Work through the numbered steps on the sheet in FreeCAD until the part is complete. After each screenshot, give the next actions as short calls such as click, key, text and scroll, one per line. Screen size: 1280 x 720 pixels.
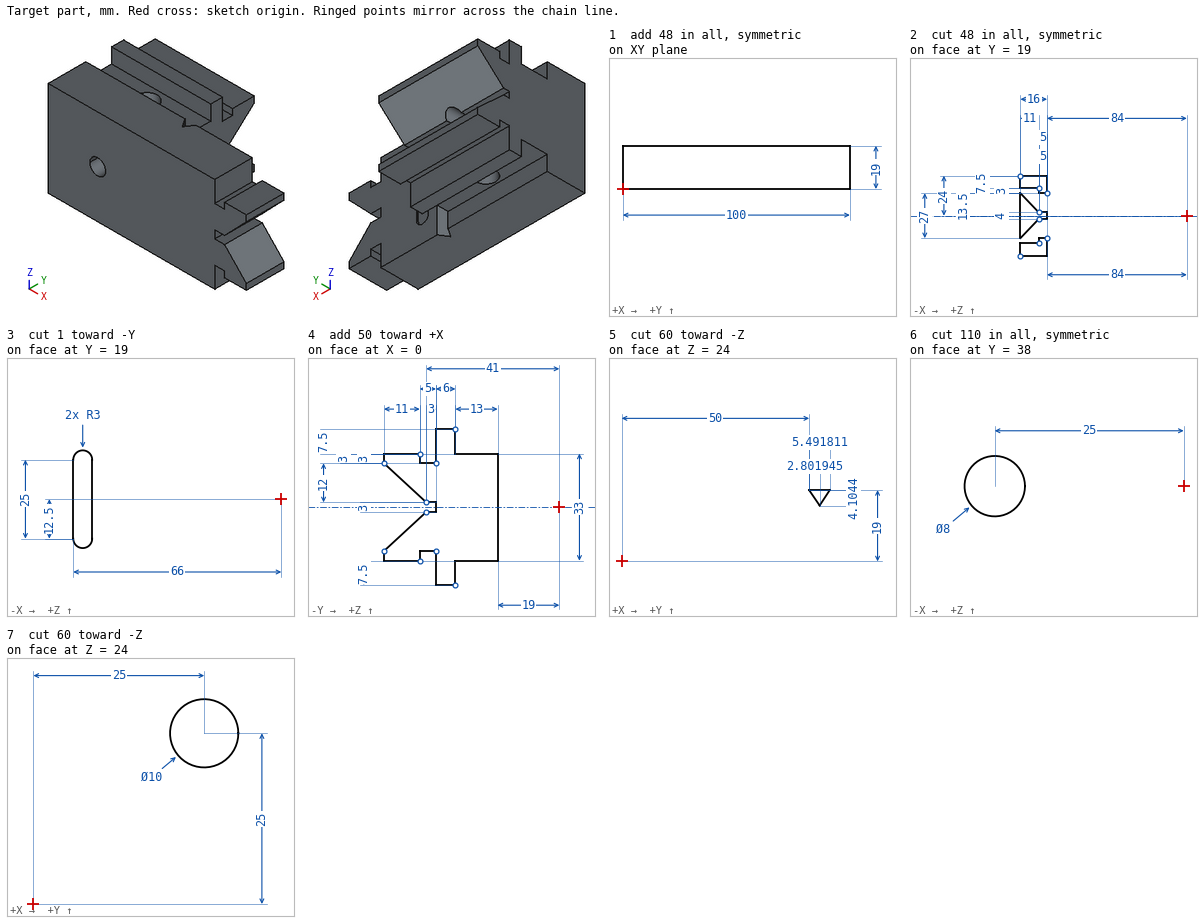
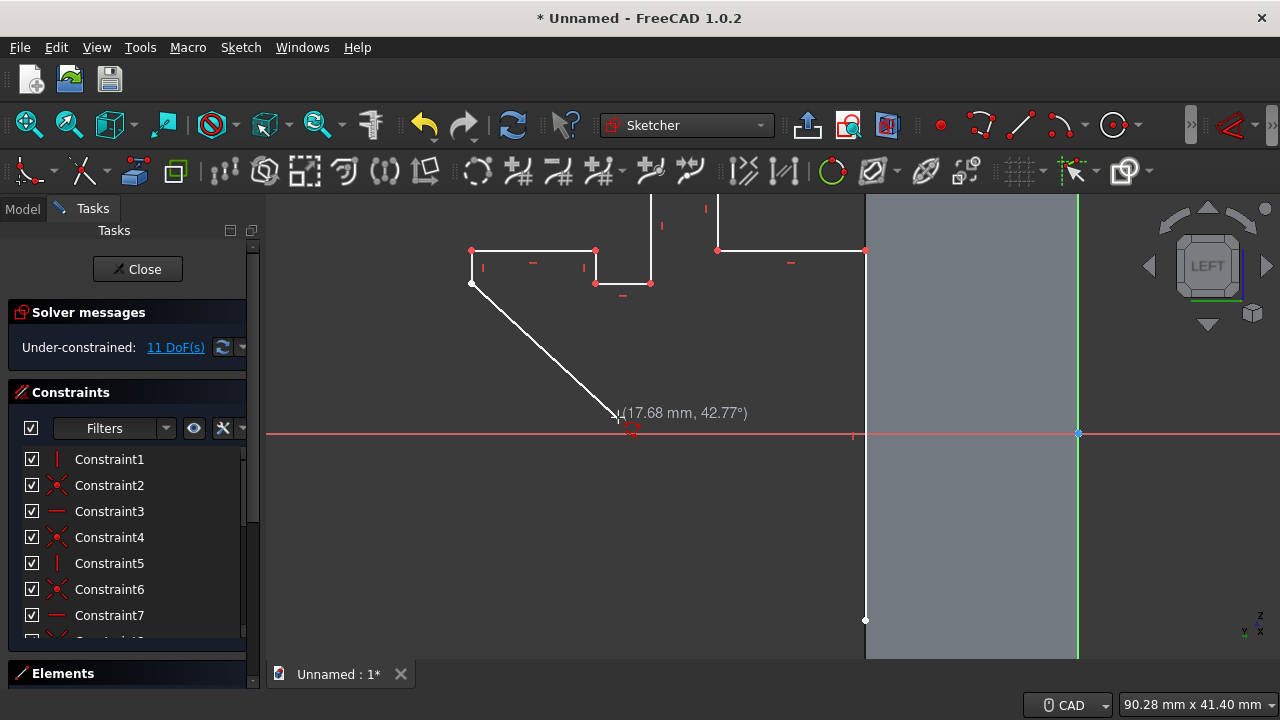
click(618, 417)
click(651, 417)
click(651, 451)
click(618, 451)
click(472, 586)
click(472, 619)
click(595, 619)
click(595, 586)
click(651, 586)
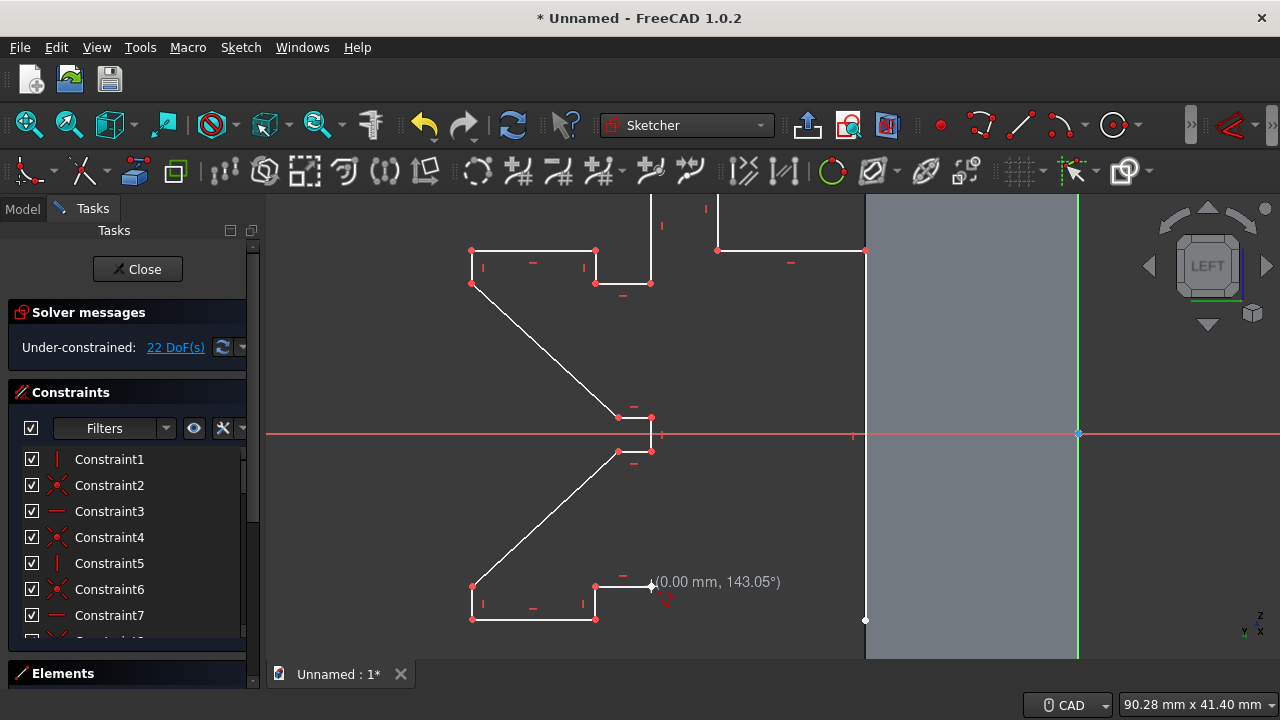
scroll(619, 417, down, 3)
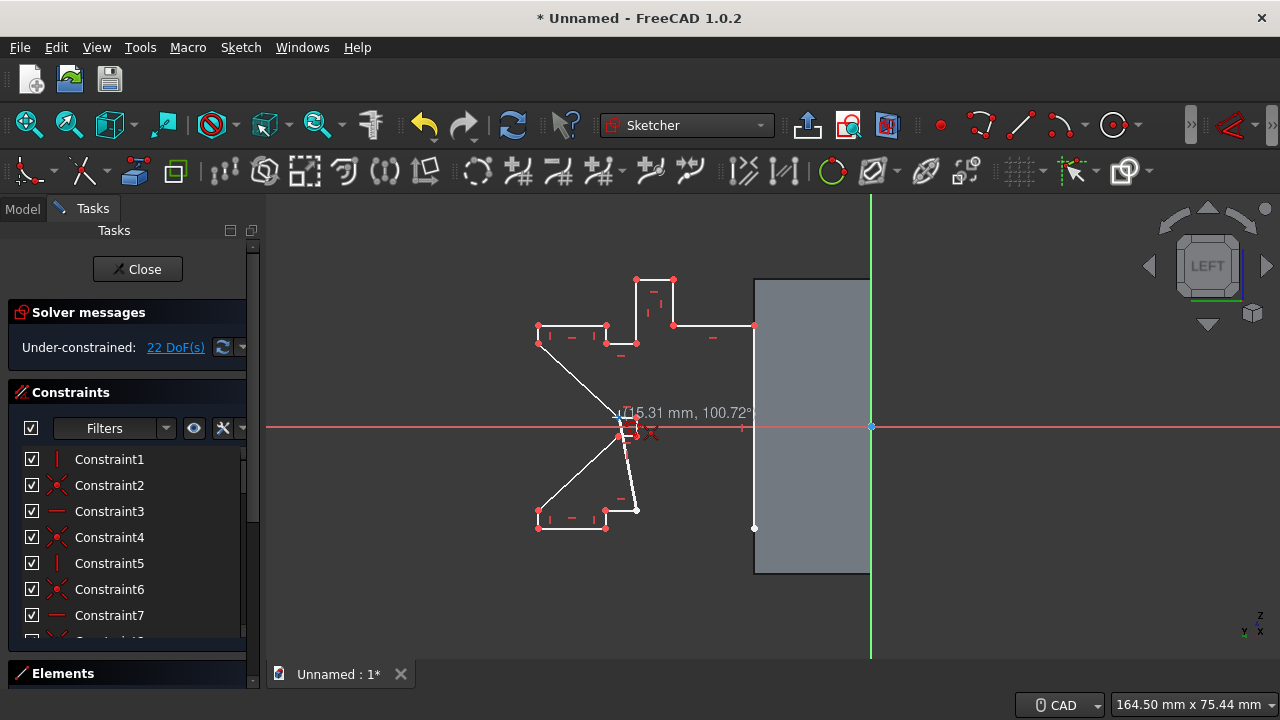
click(637, 574)
click(674, 574)
click(674, 528)
click(754, 529)
key(Escape)
key(Escape)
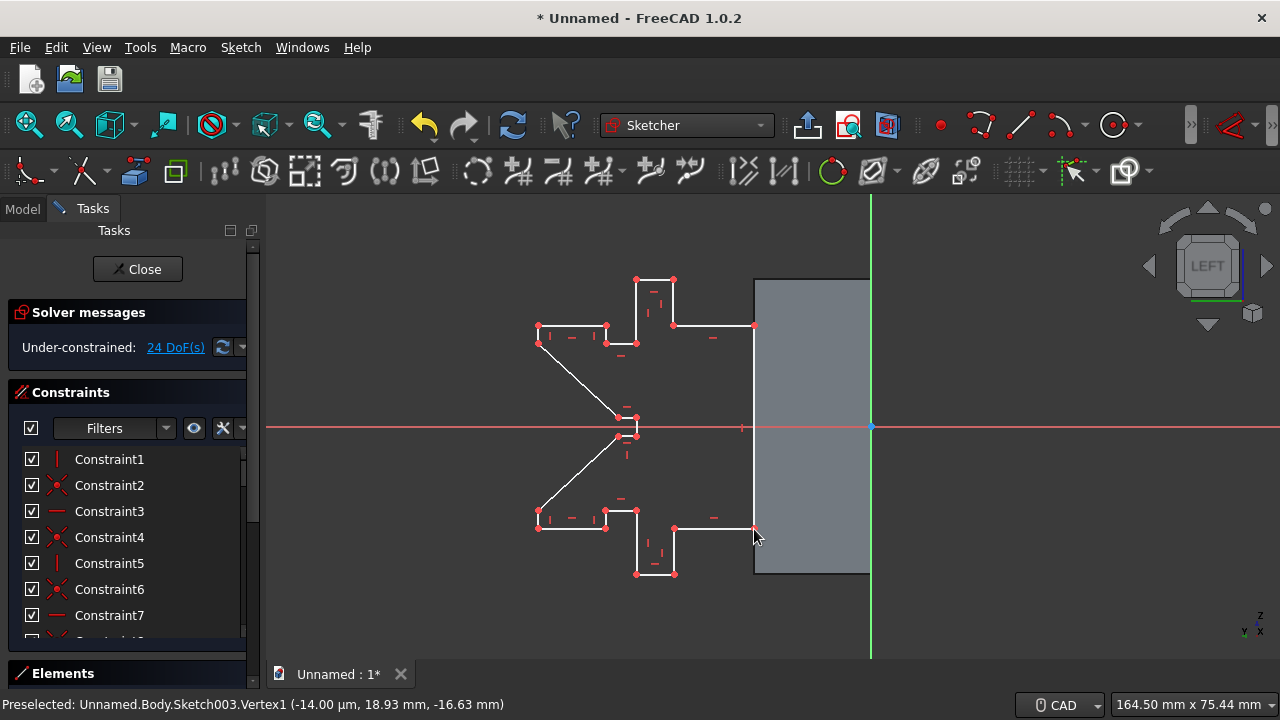
click(619, 418)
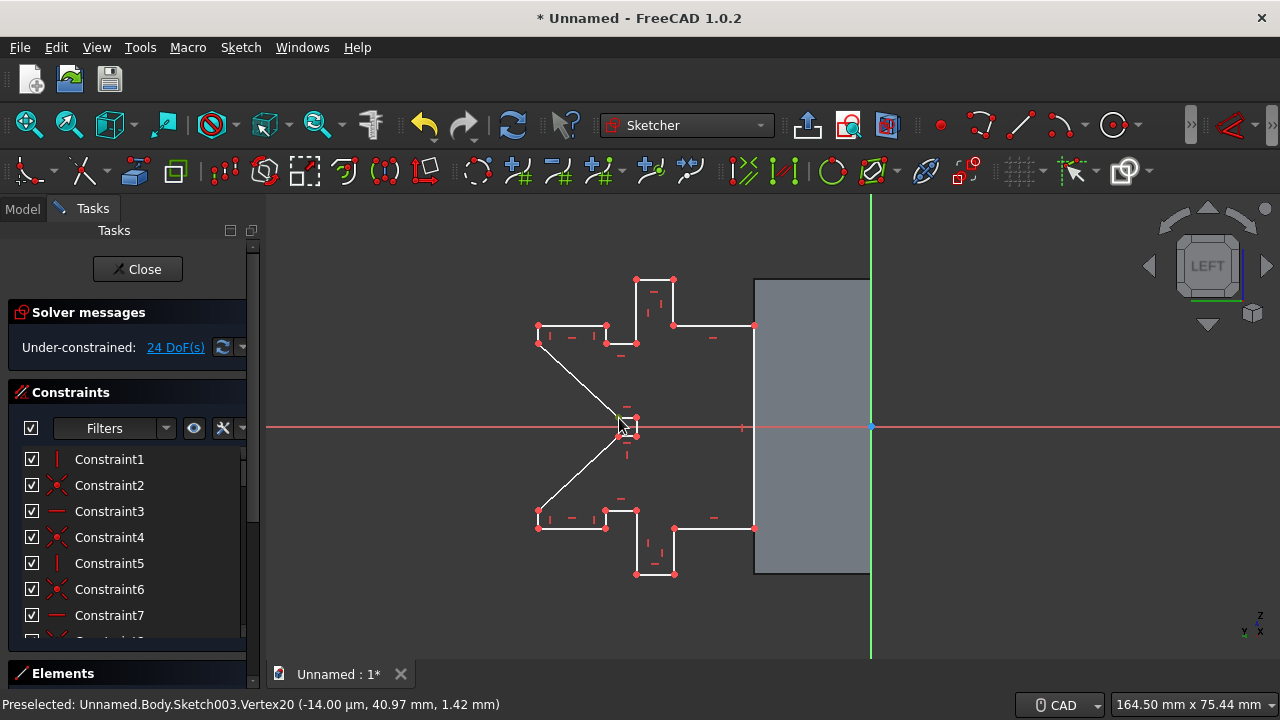
click(619, 436)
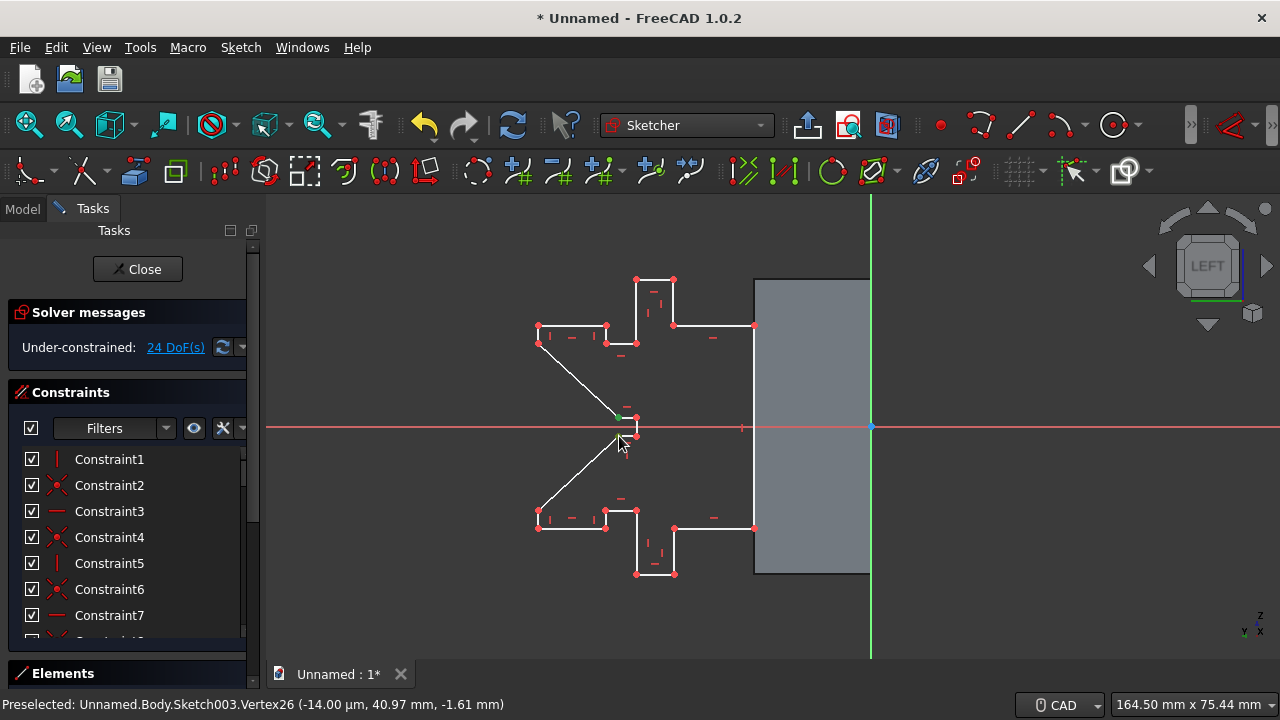
click(353, 426)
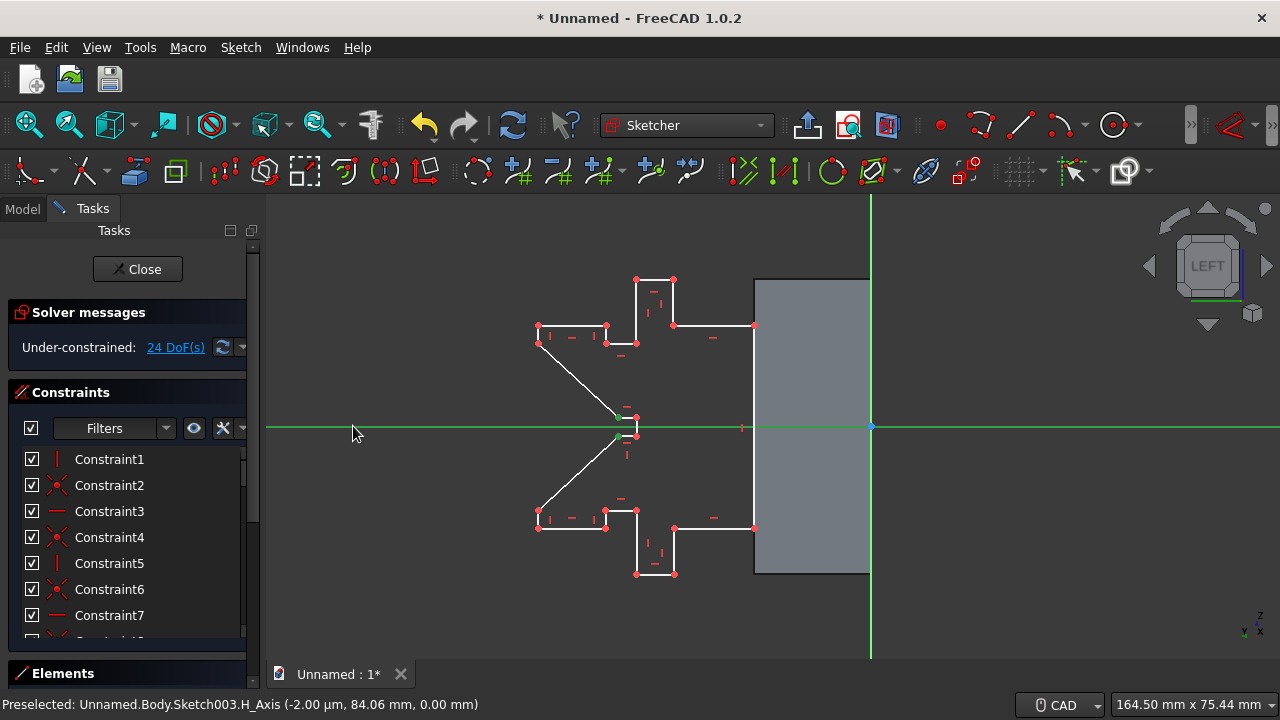
key(s)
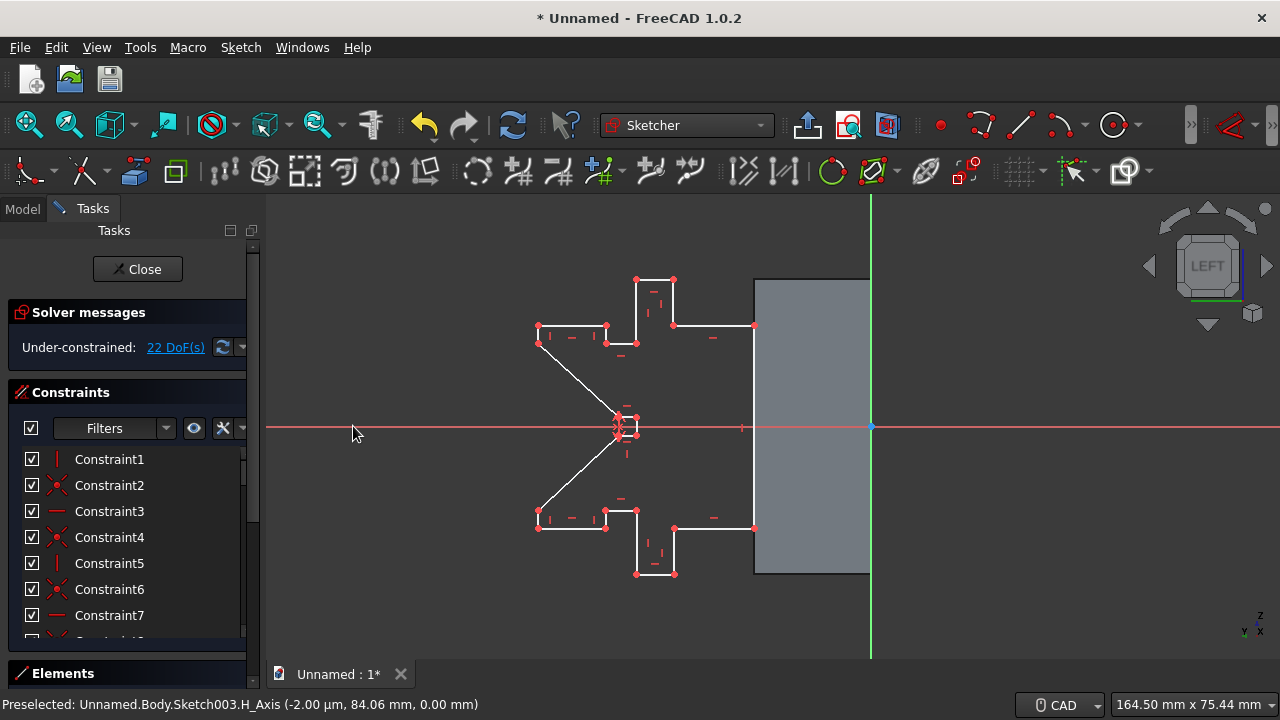
click(538, 344)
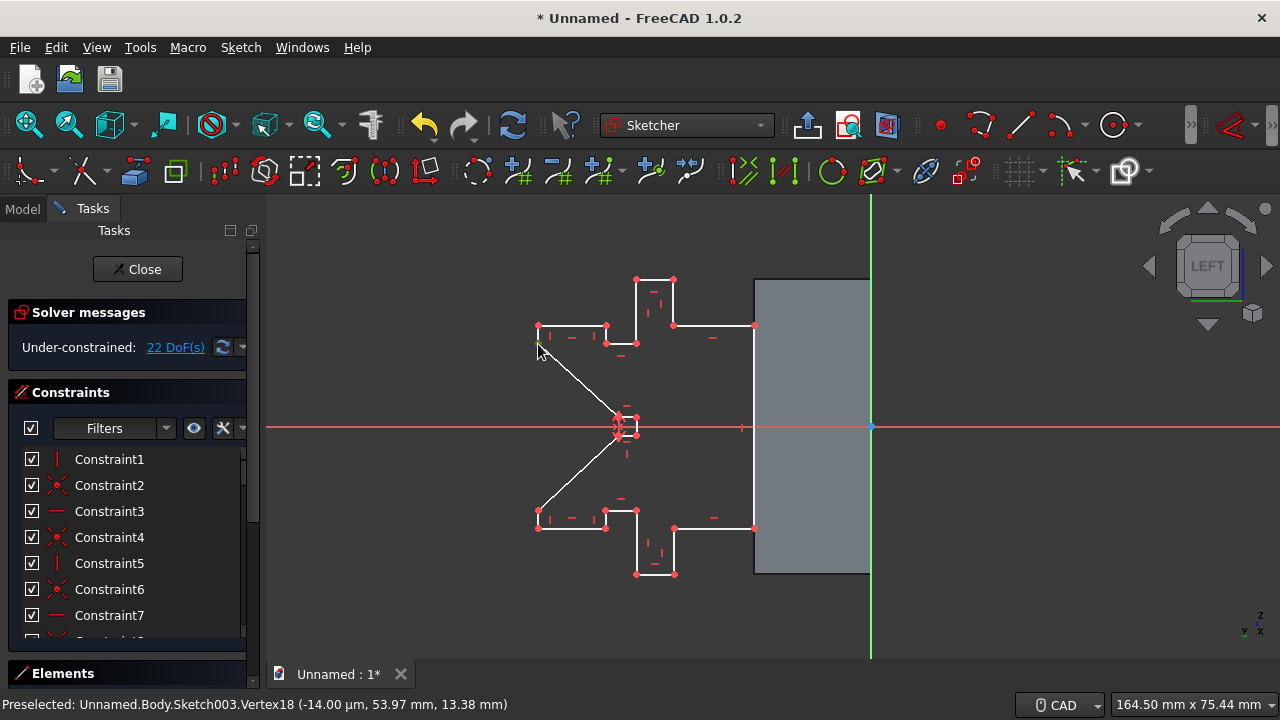
click(538, 511)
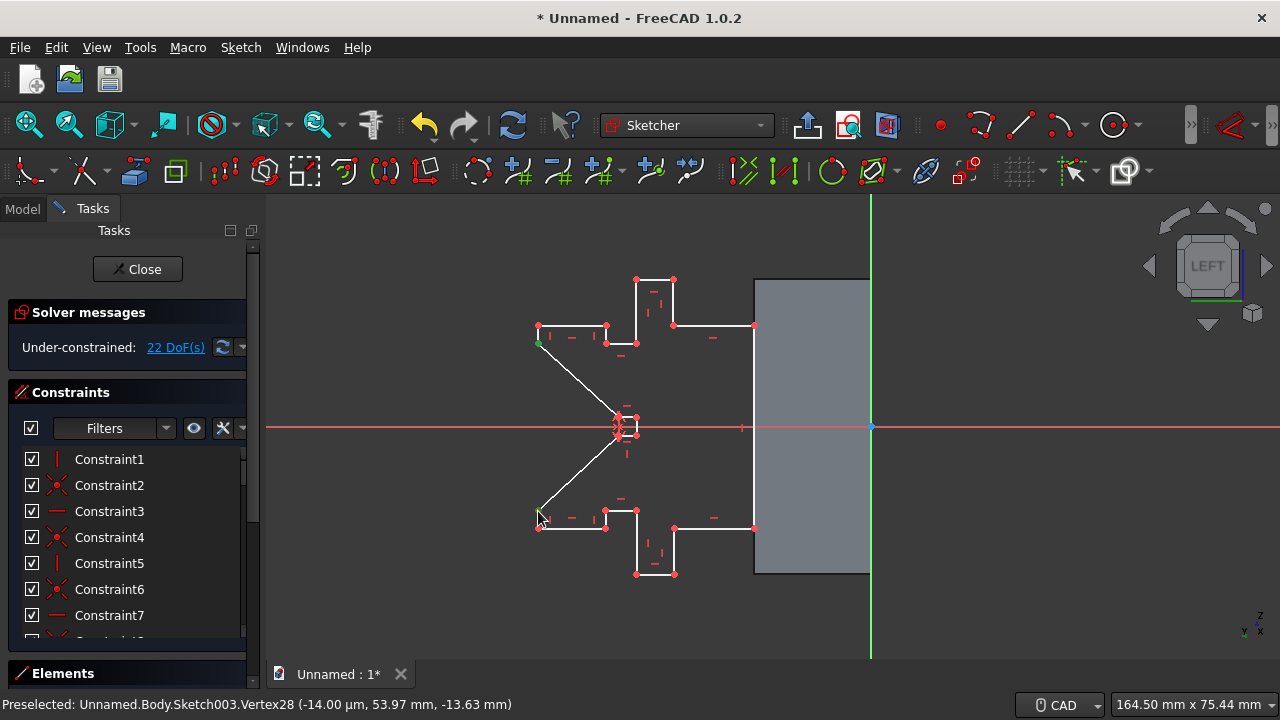
click(353, 426)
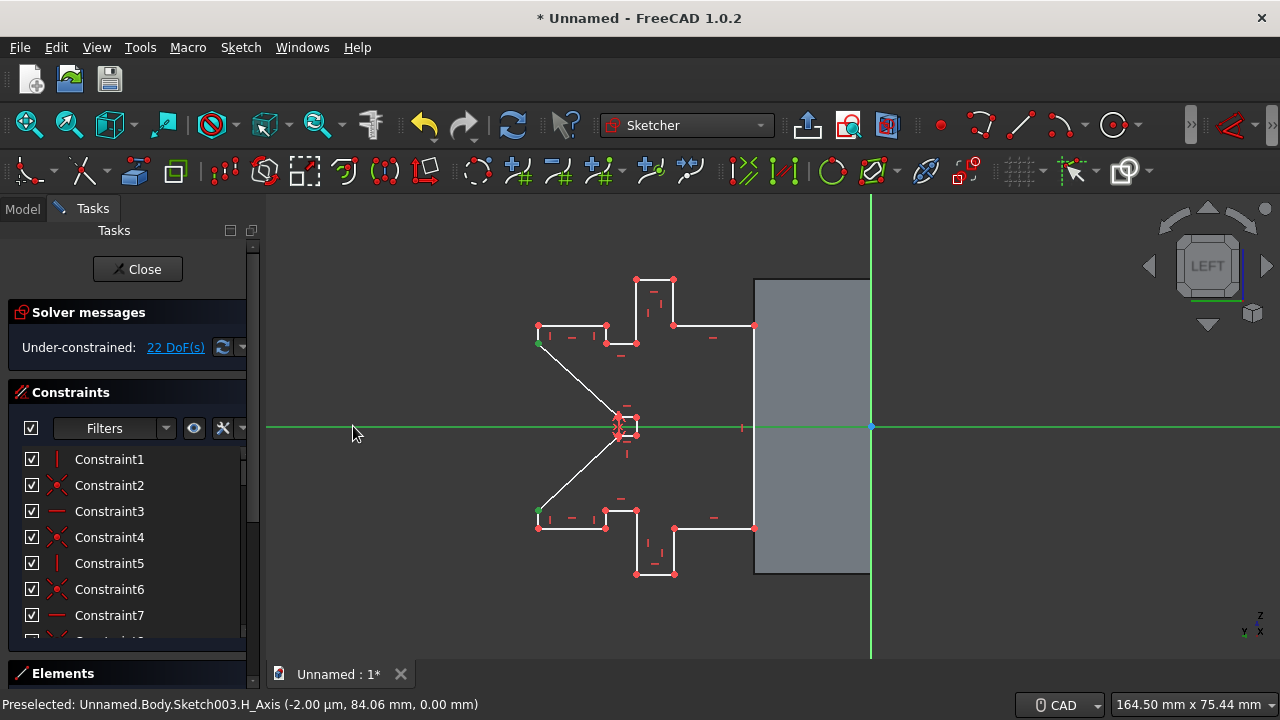
key(s)